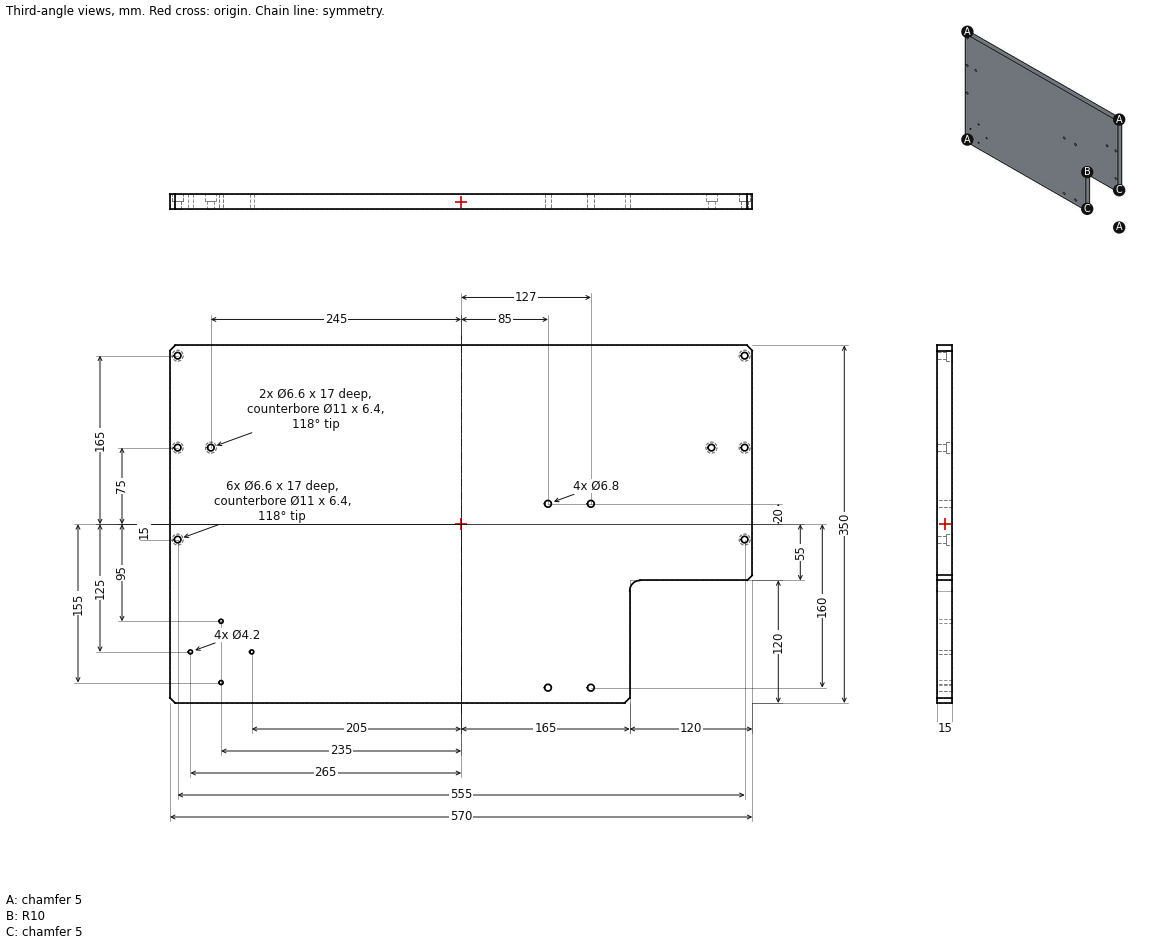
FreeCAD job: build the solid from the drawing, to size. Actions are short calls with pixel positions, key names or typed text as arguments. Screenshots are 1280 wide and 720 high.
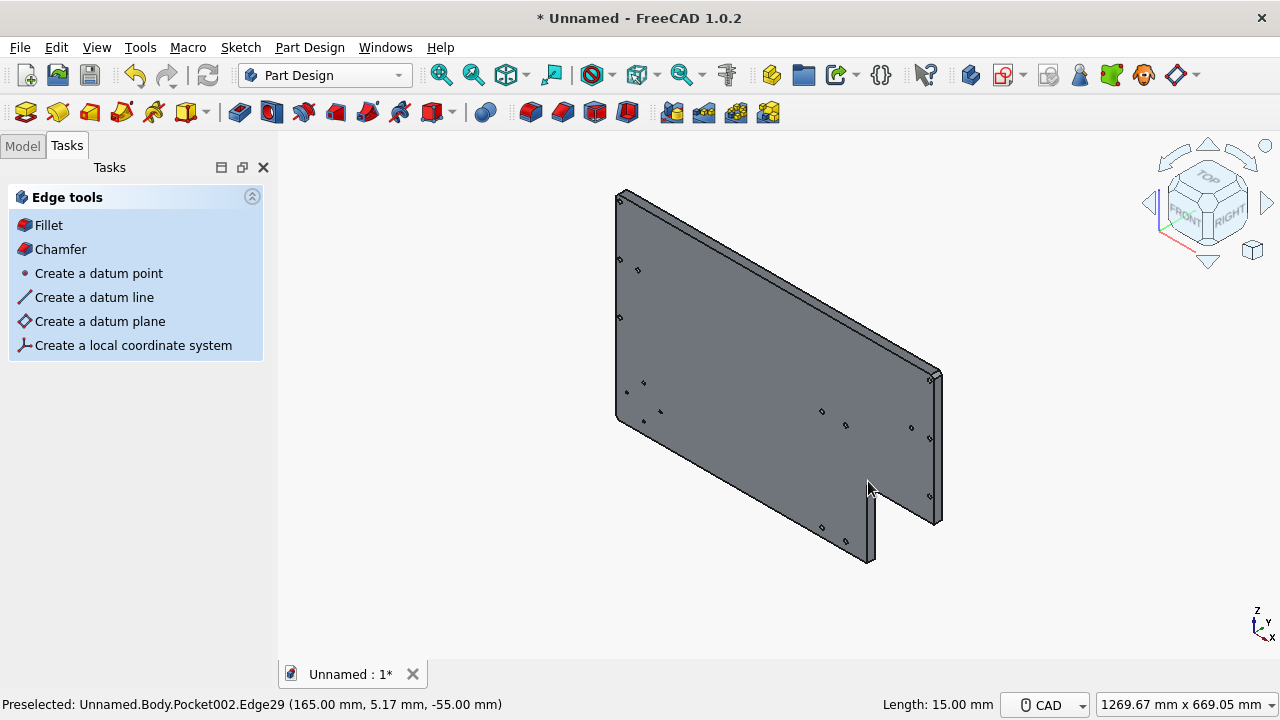
click(532, 112)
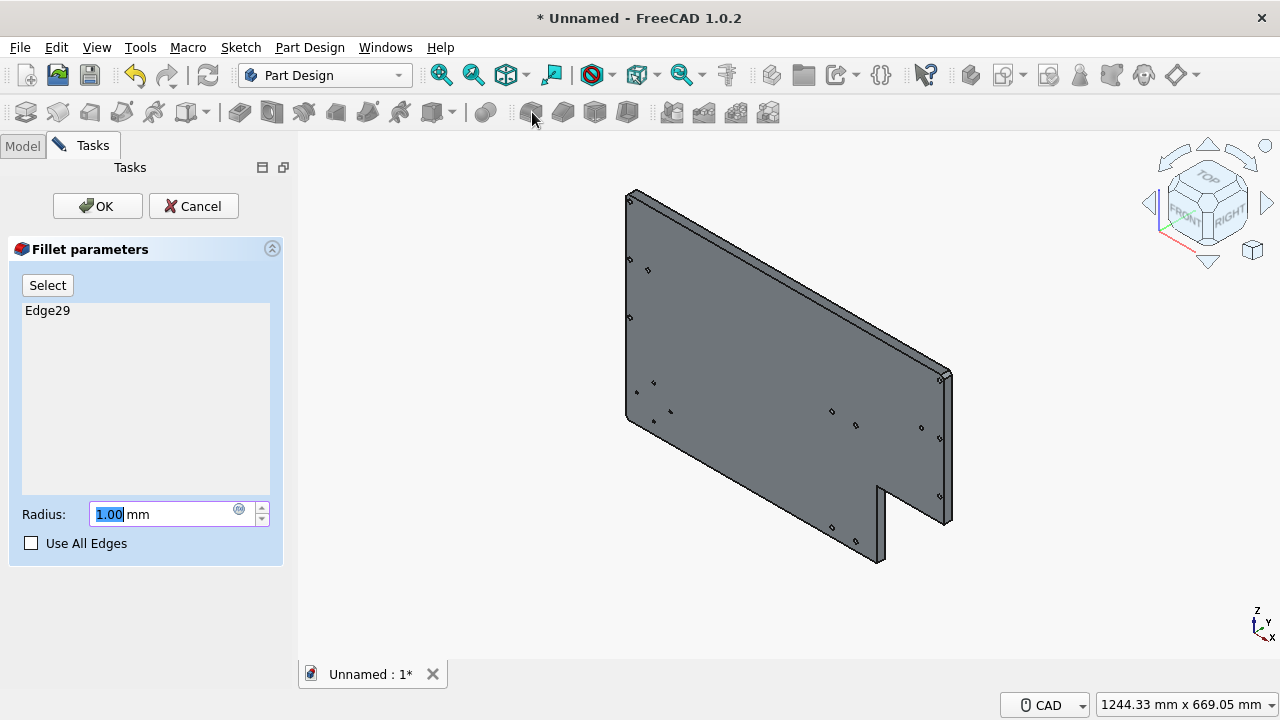
text(10)
key(Tab)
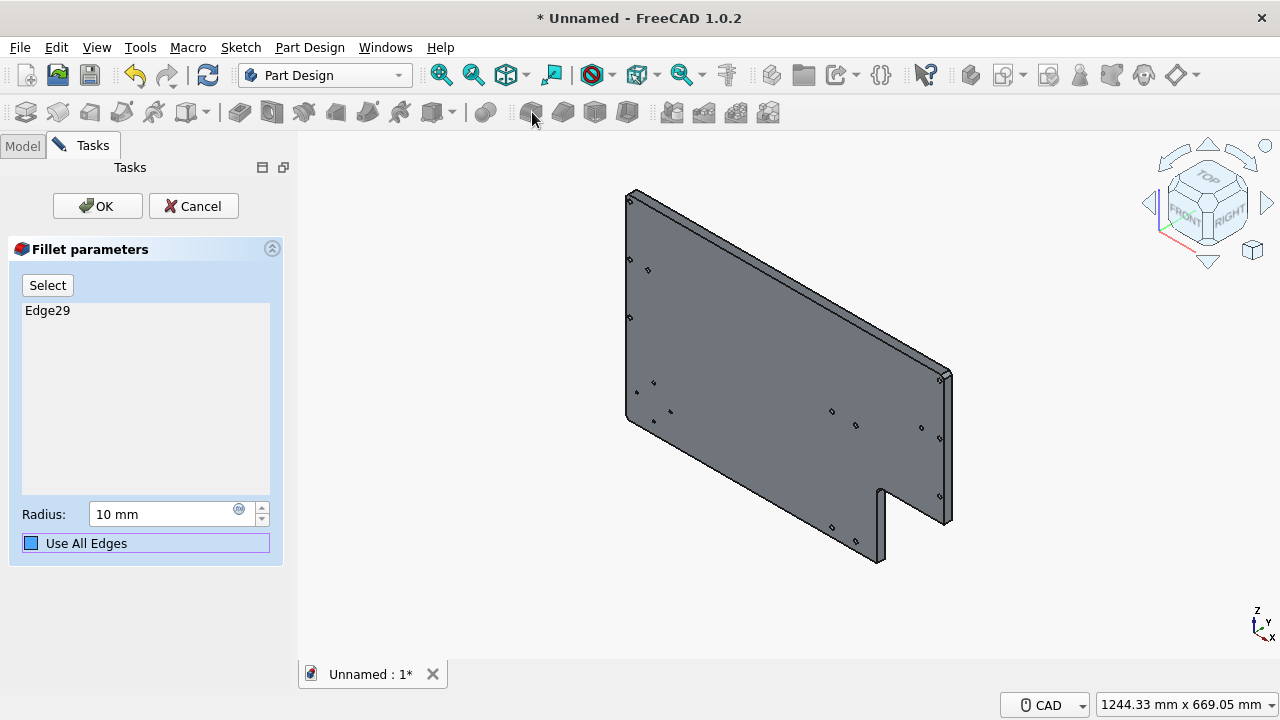
click(98, 206)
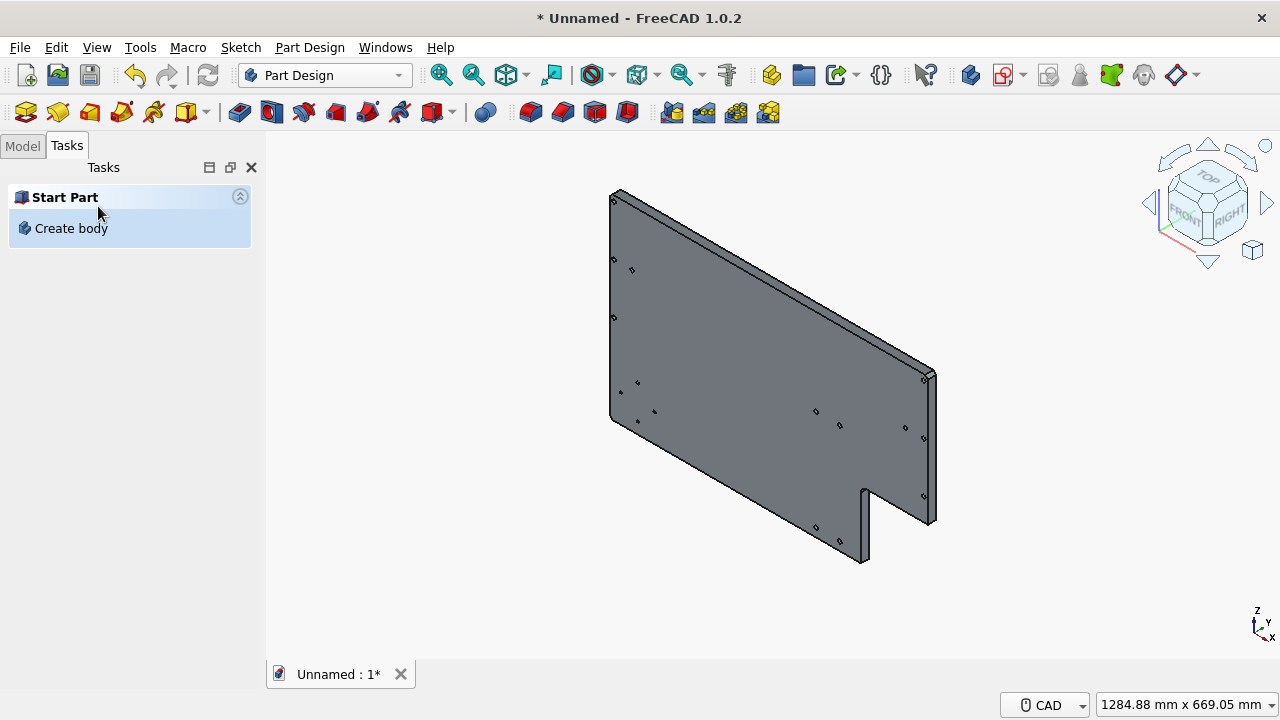
scroll(932, 521, up, 7)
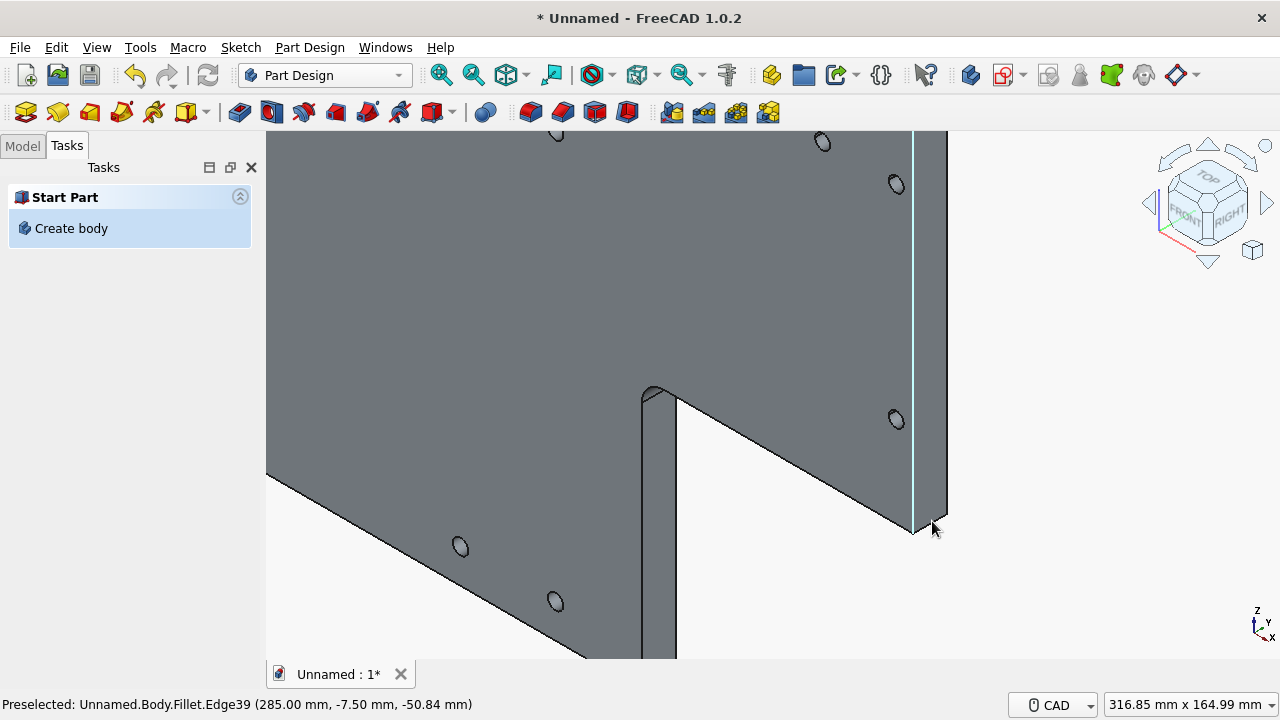
click(442, 76)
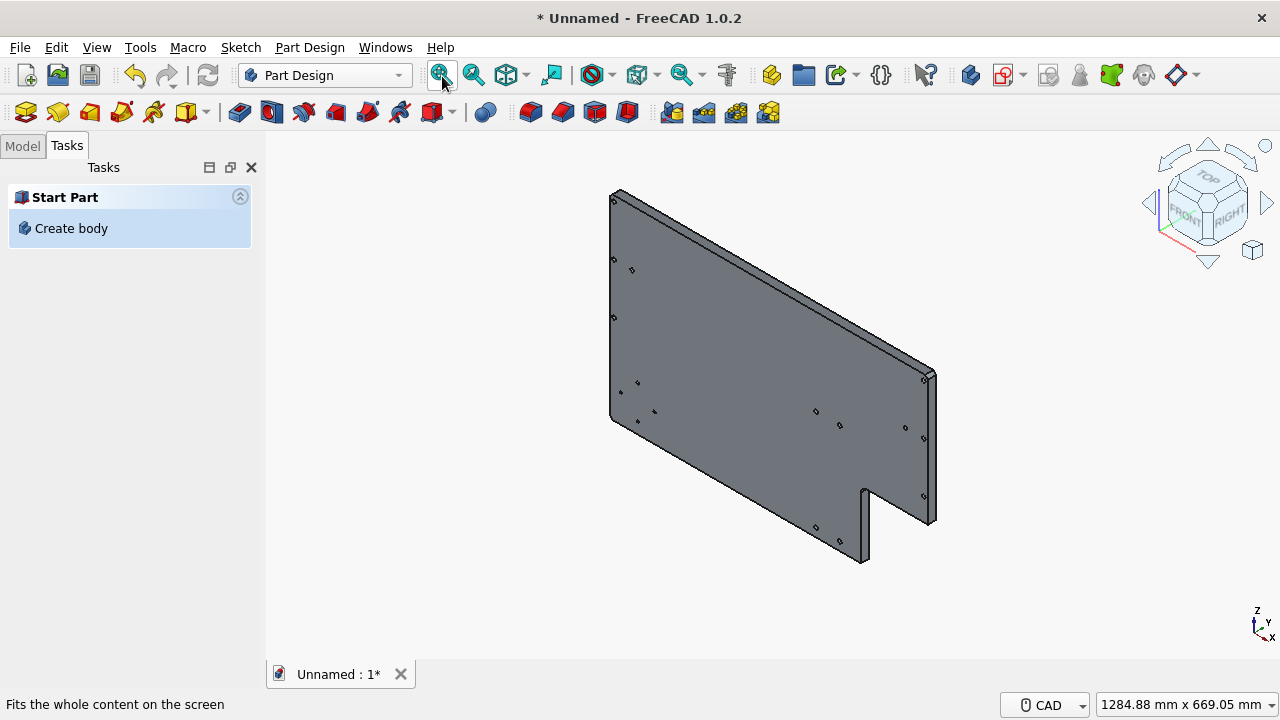
key(2)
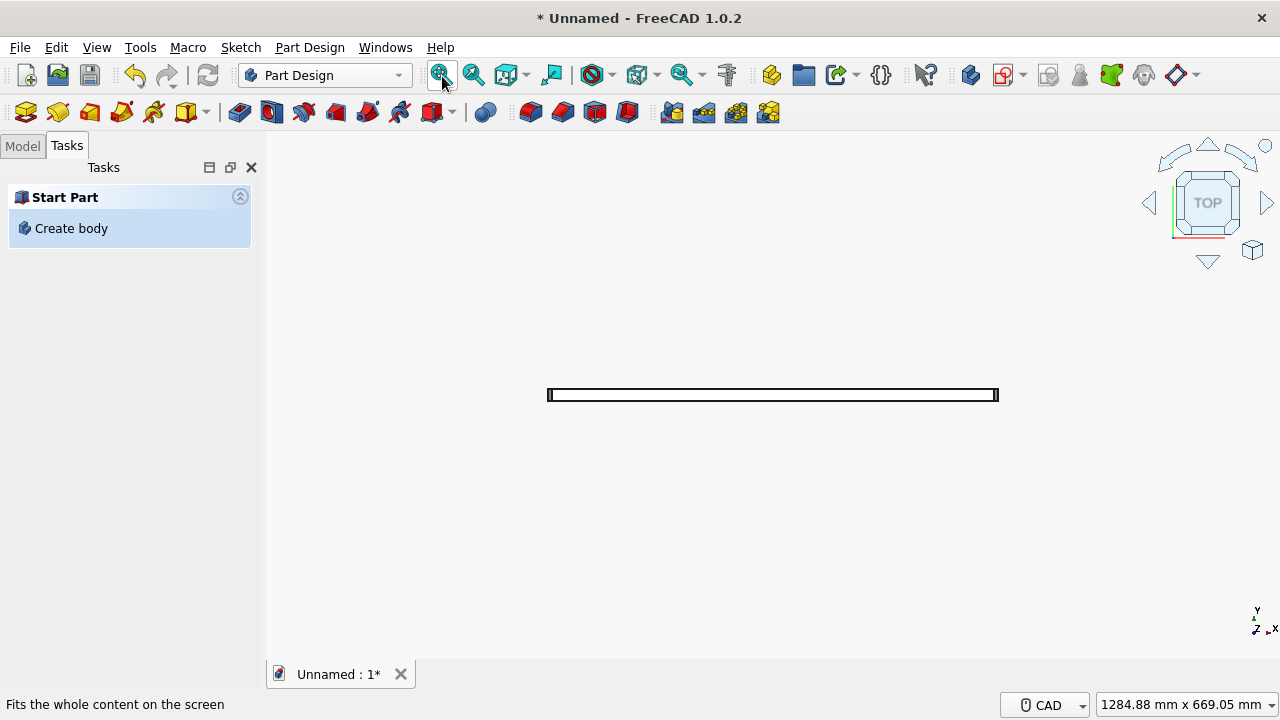
click(442, 76)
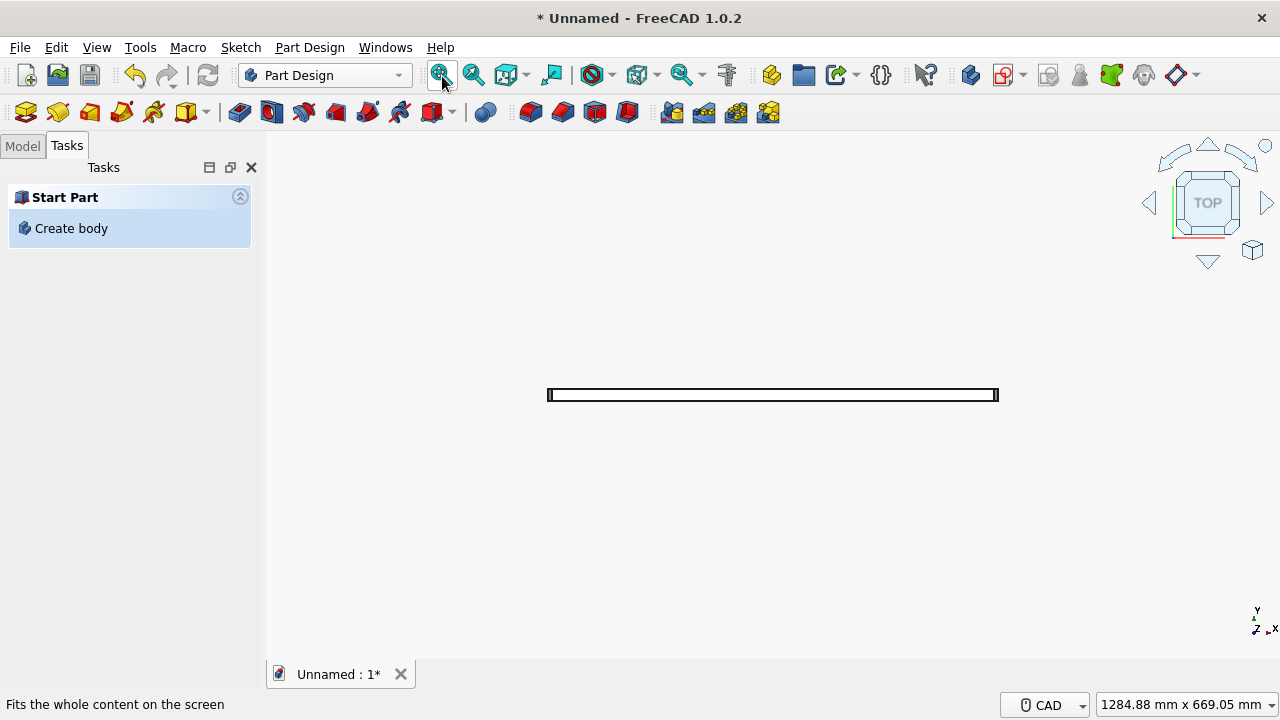
scroll(998, 394, up, 7)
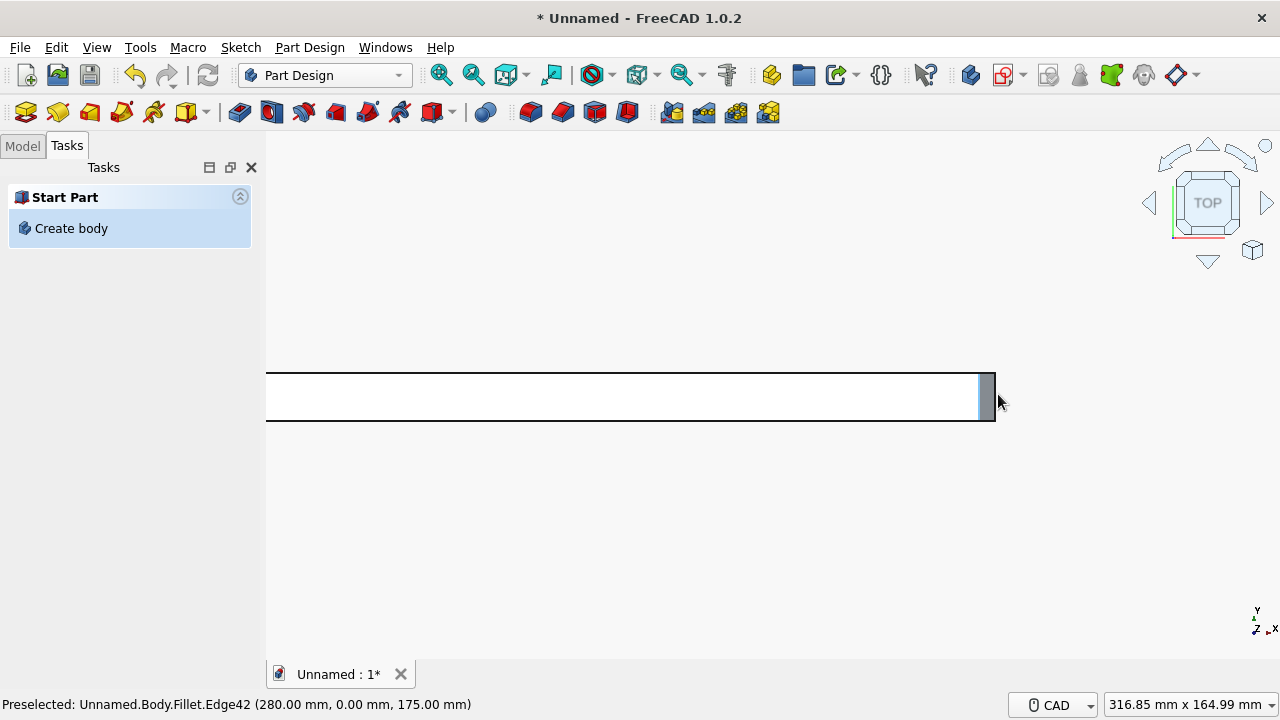
click(442, 76)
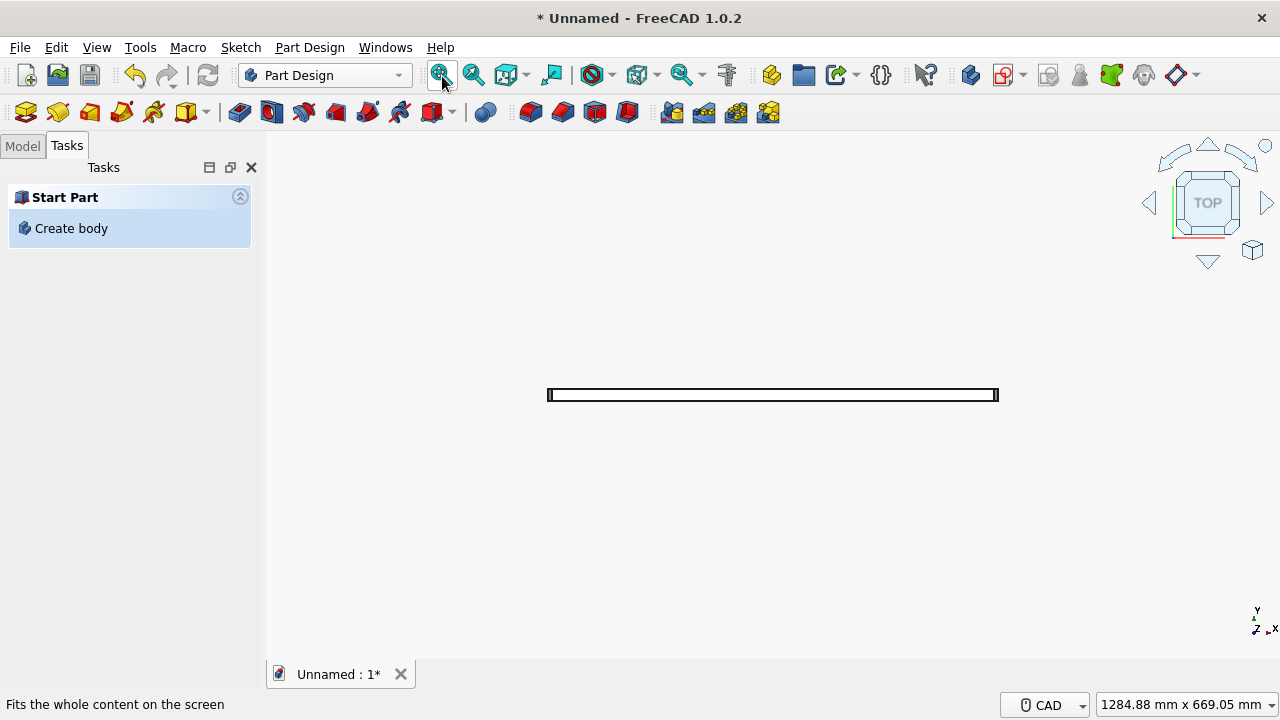
key(0)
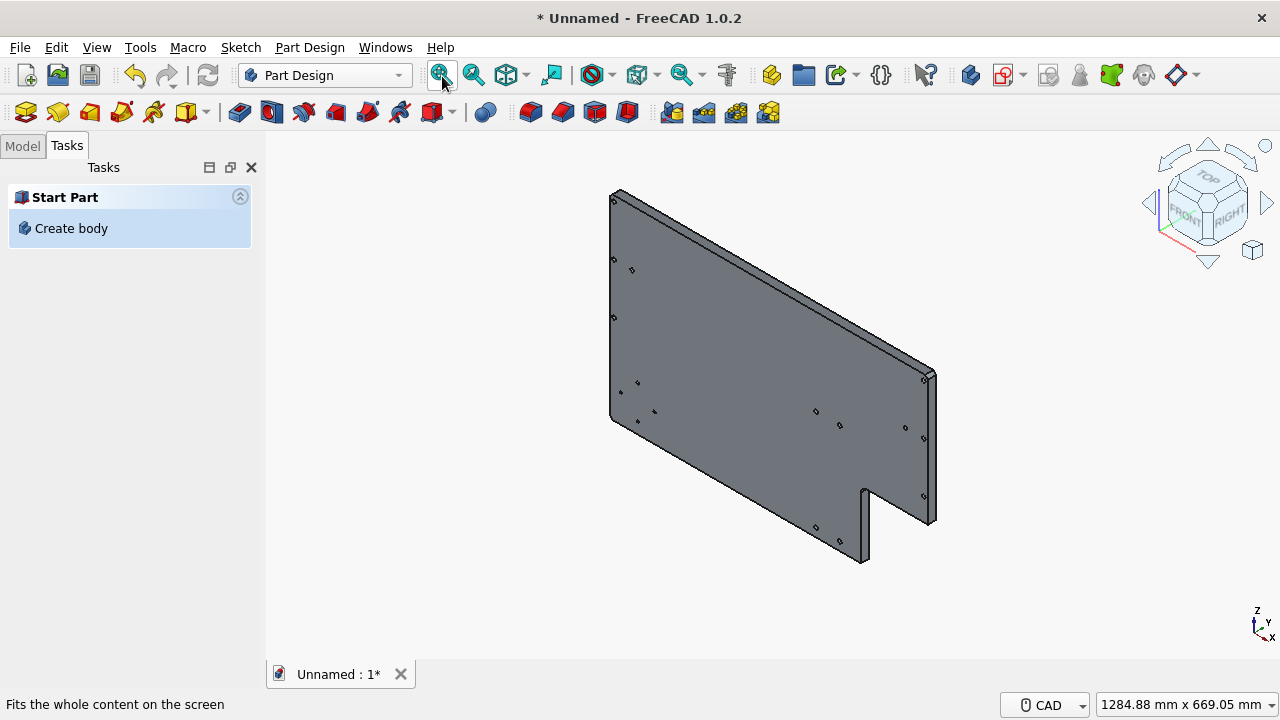
scroll(932, 521, up, 7)